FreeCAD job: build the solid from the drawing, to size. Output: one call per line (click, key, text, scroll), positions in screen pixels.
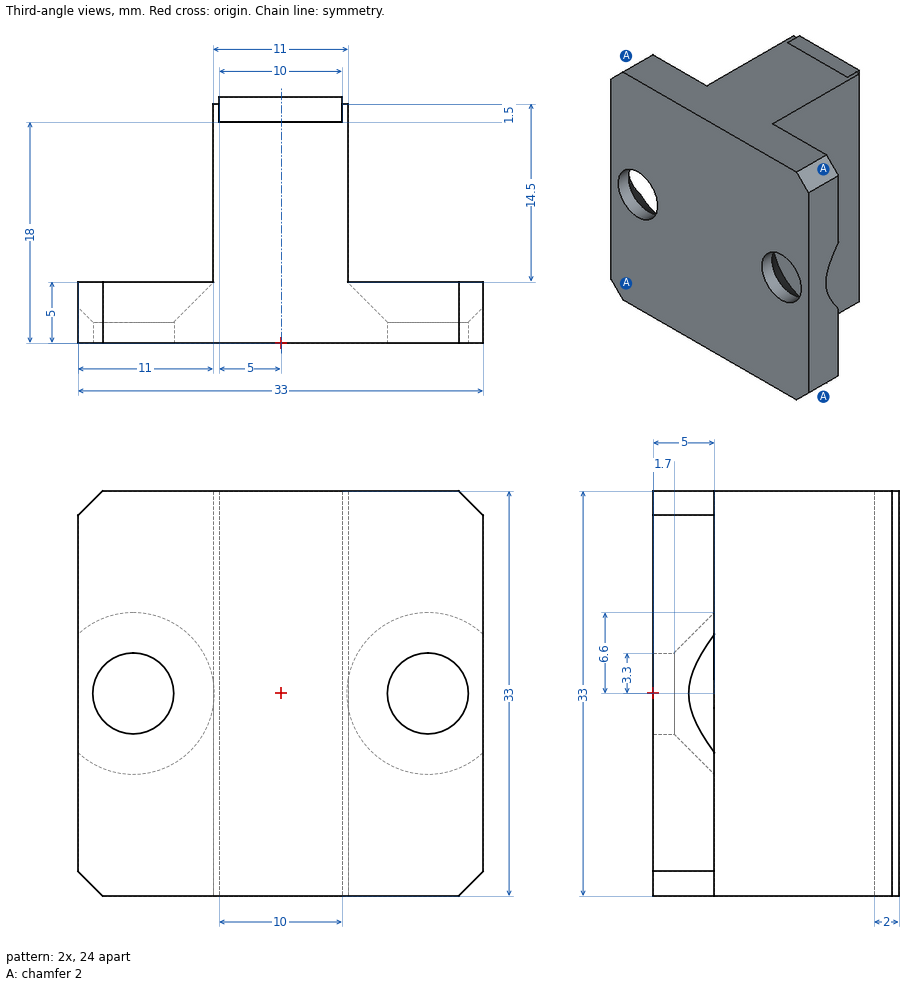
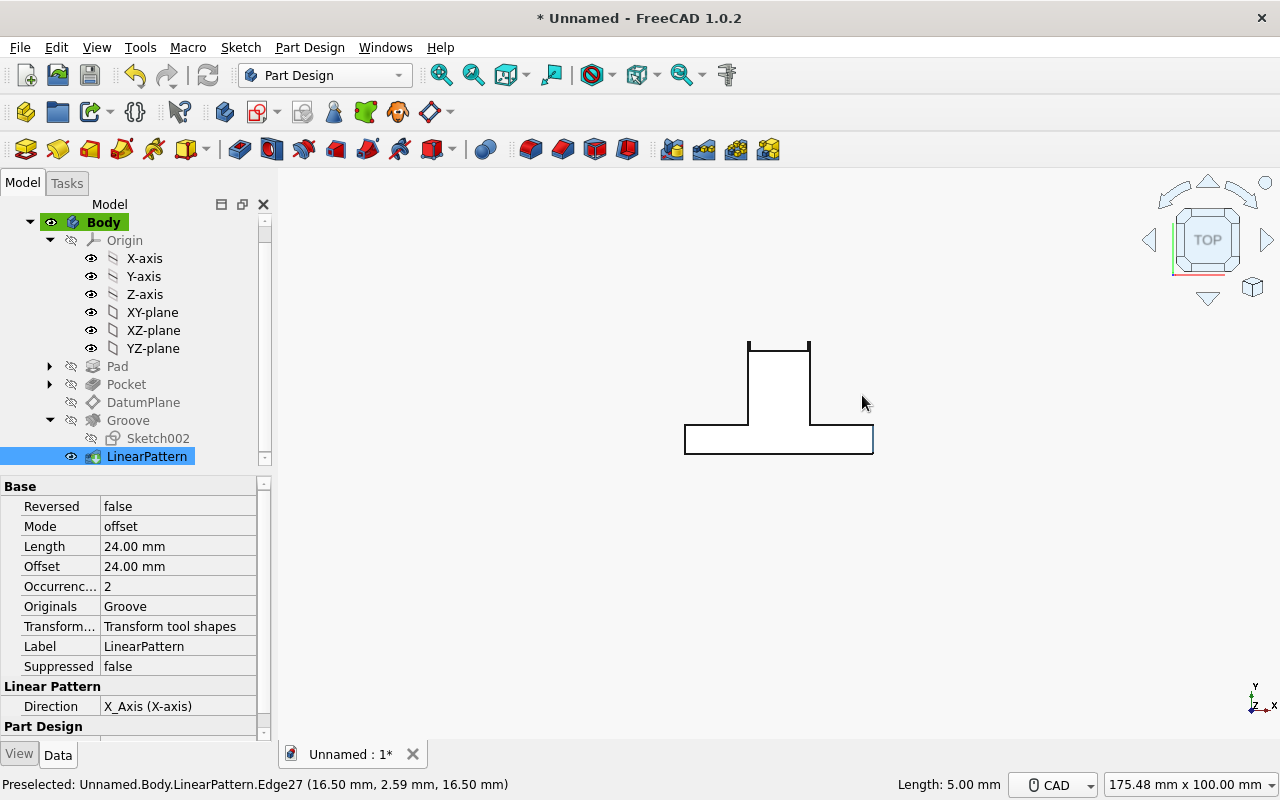
click(442, 76)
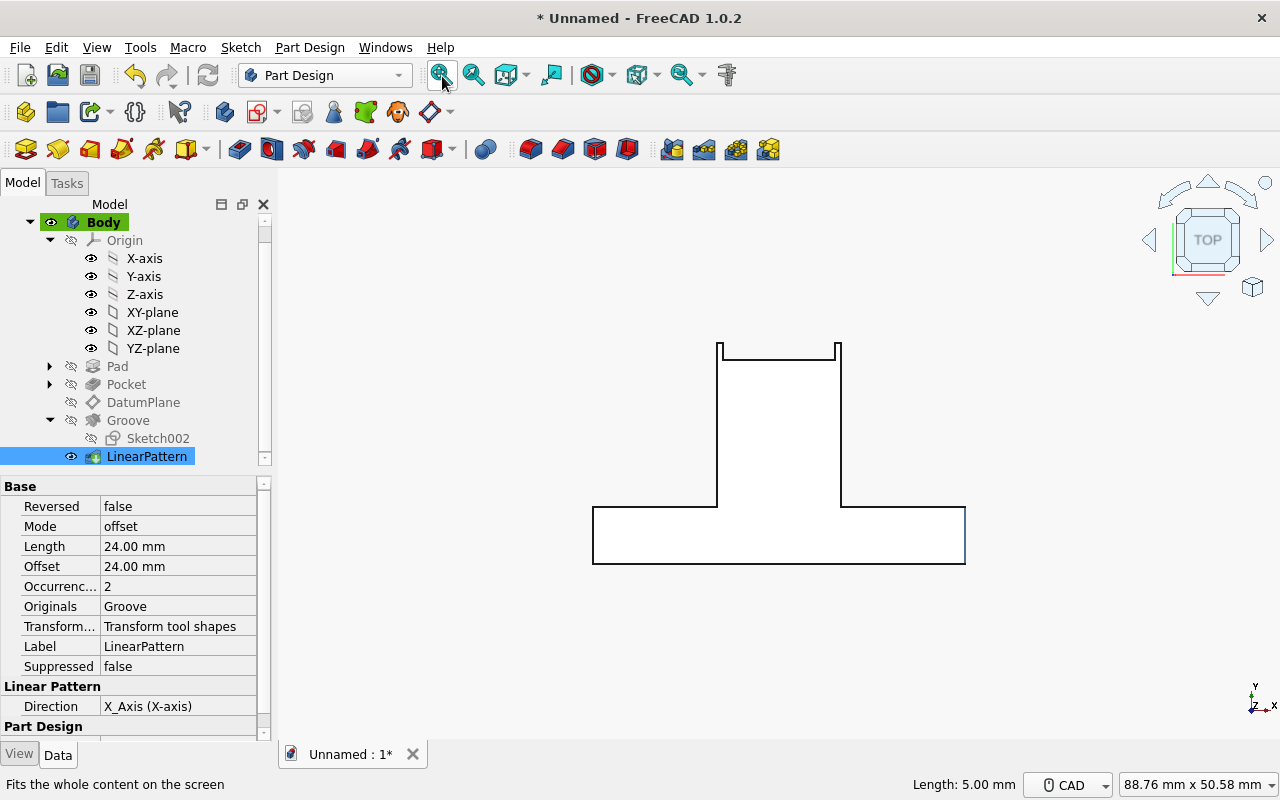
click(593, 534, ctrl)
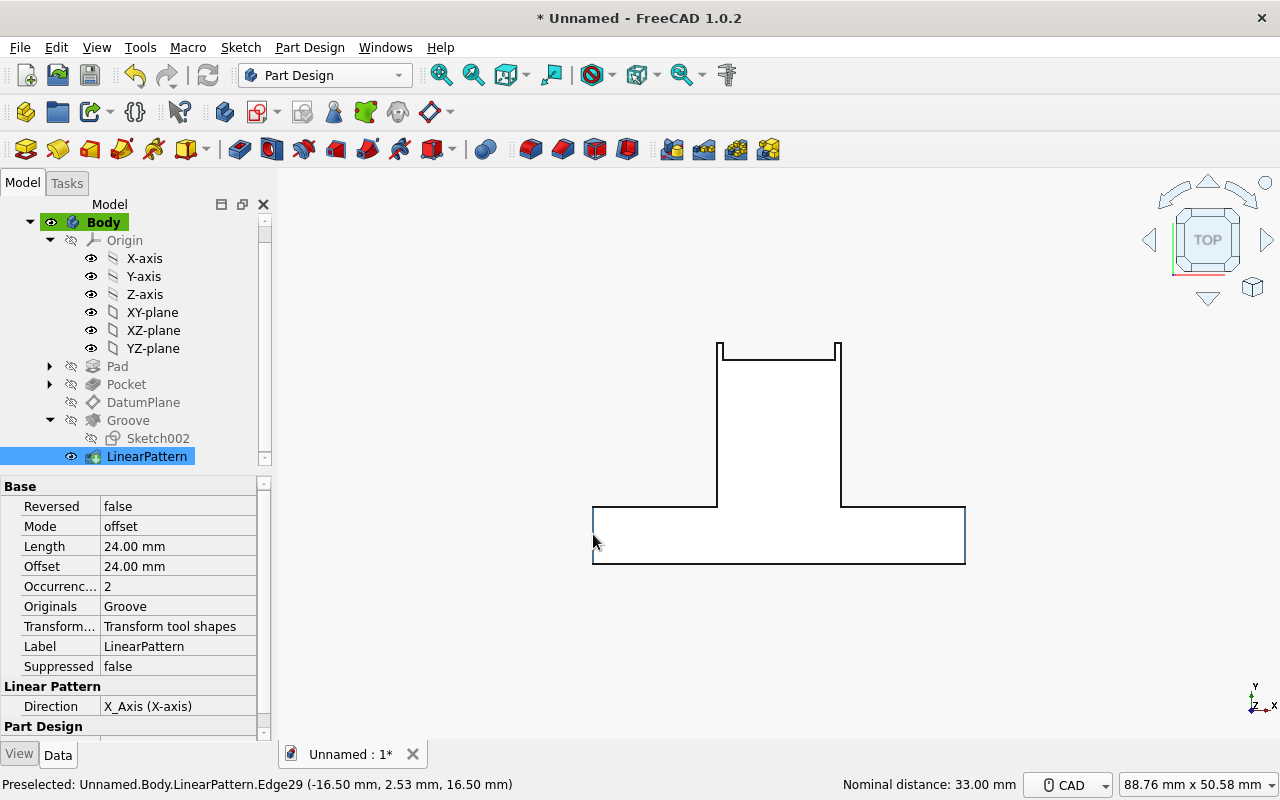
key(1)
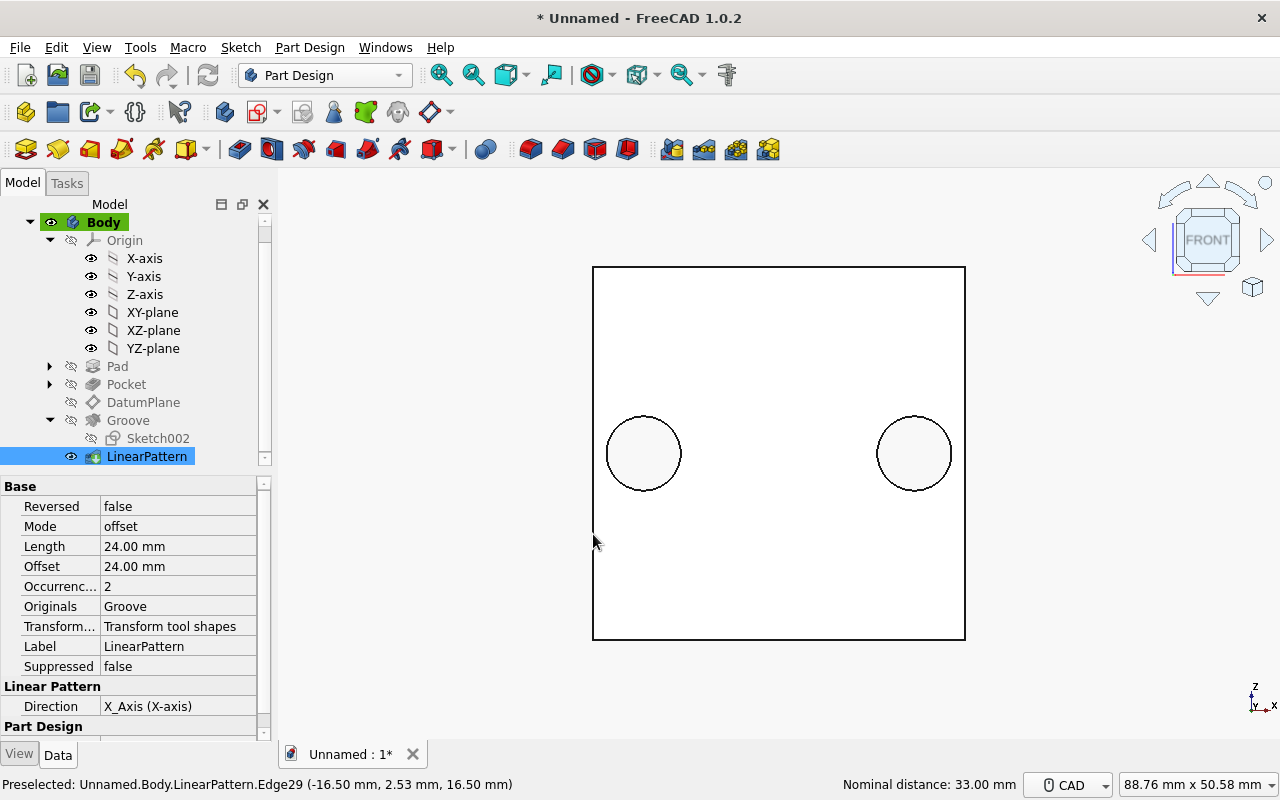
key(3)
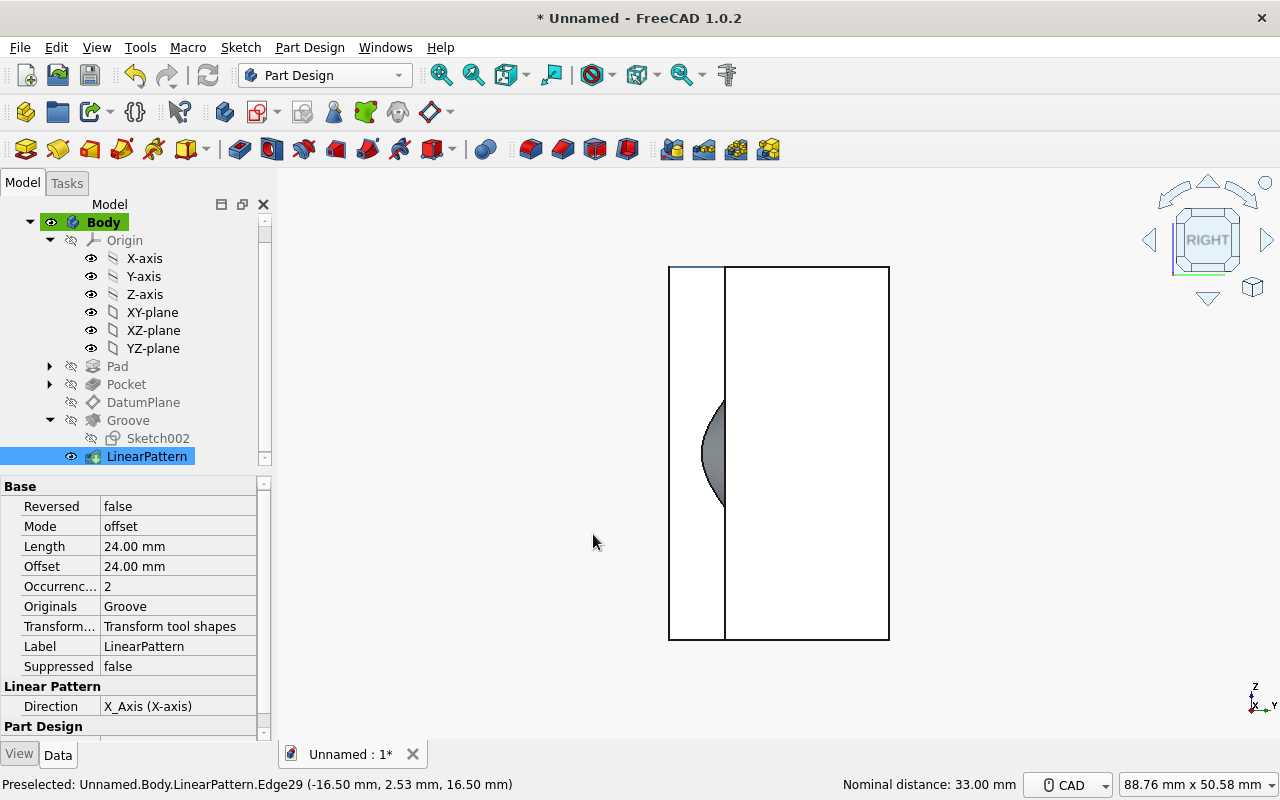
click(697, 639, ctrl)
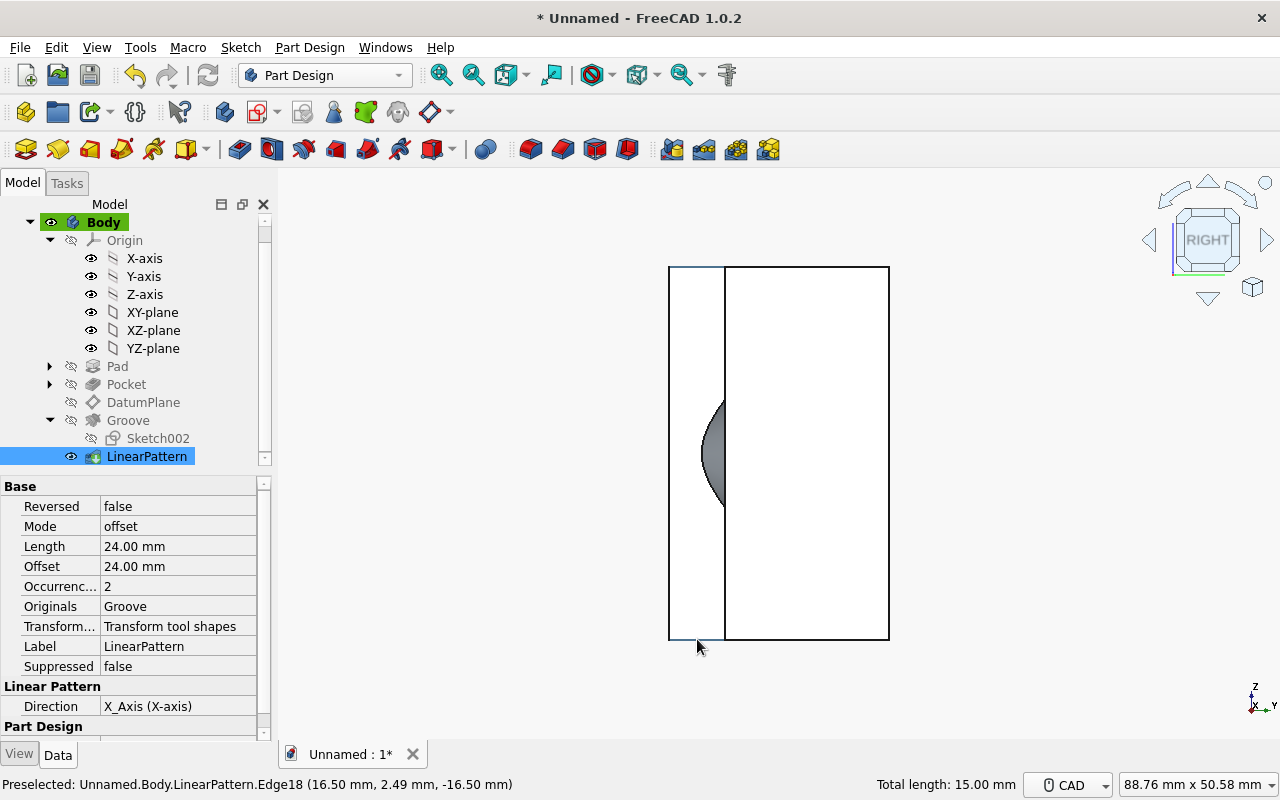
key(5)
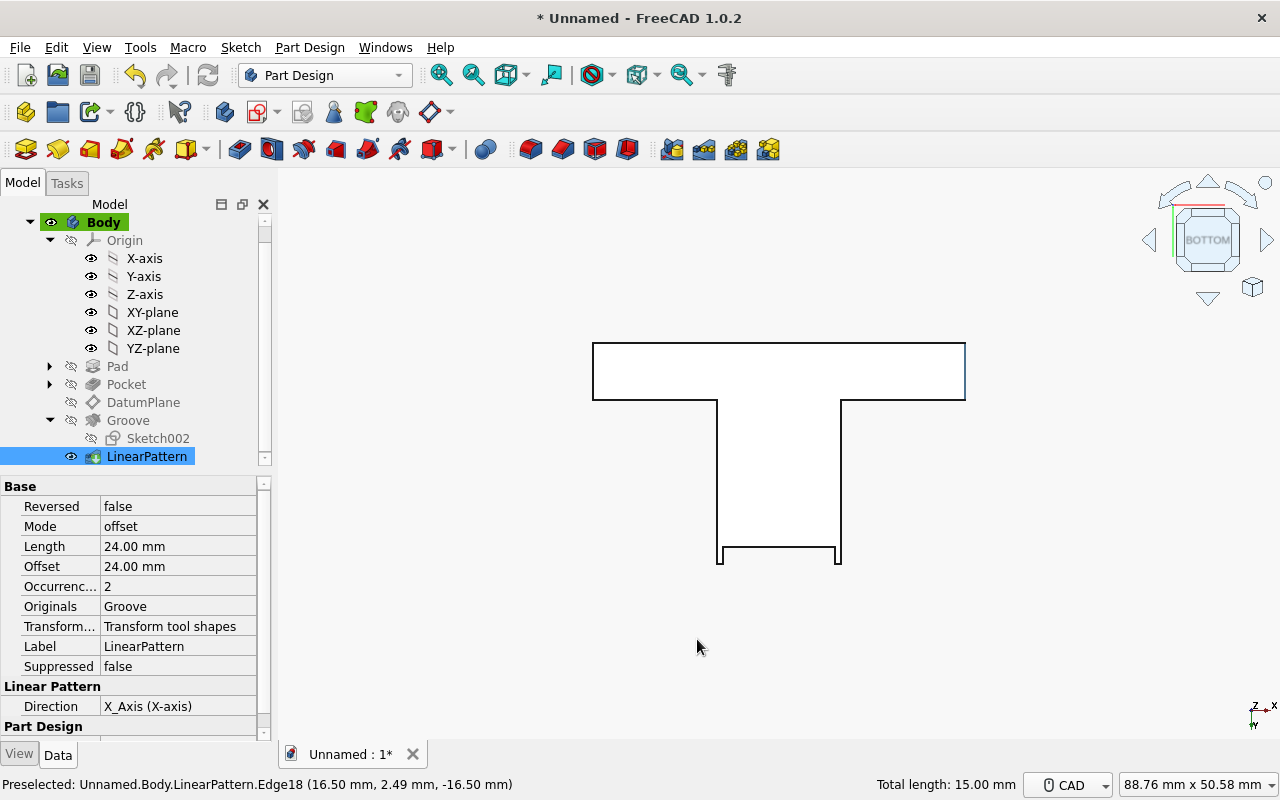
key(v)
key(f)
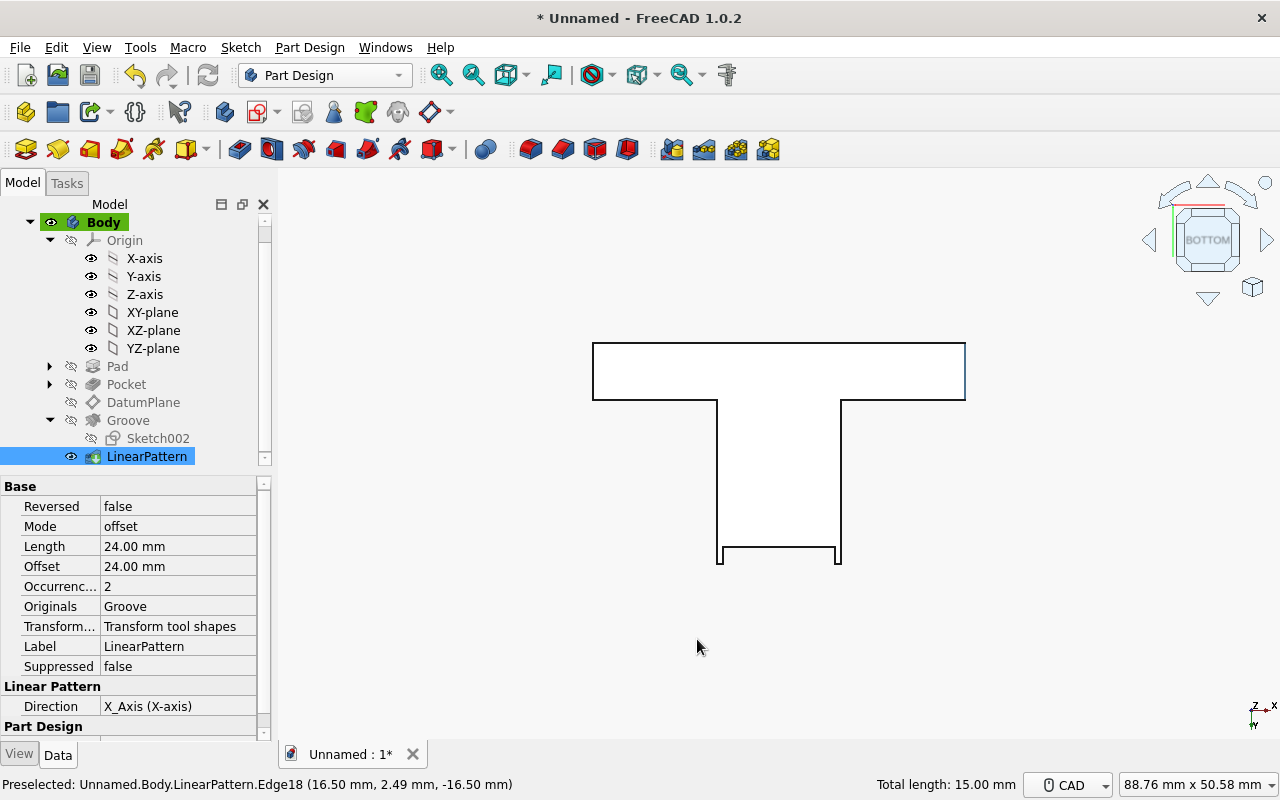
click(593, 371, ctrl)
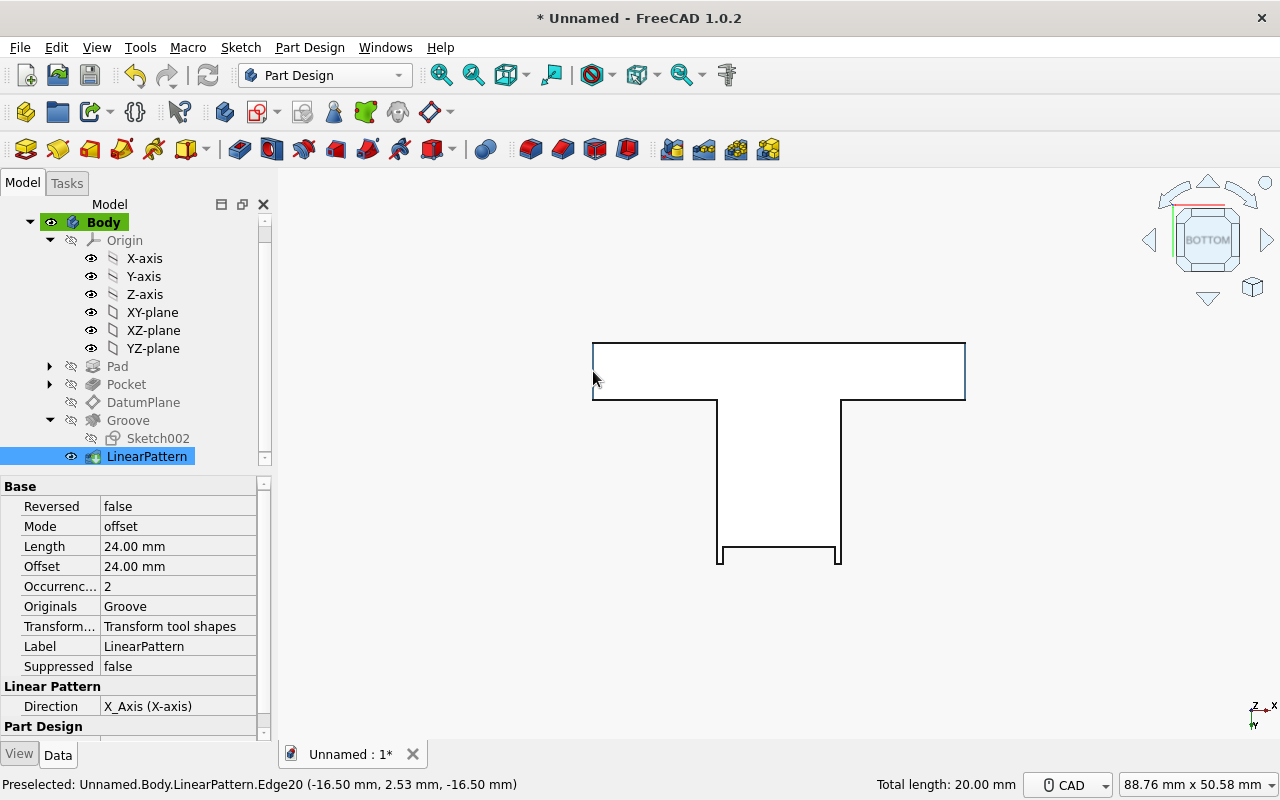
click(564, 150)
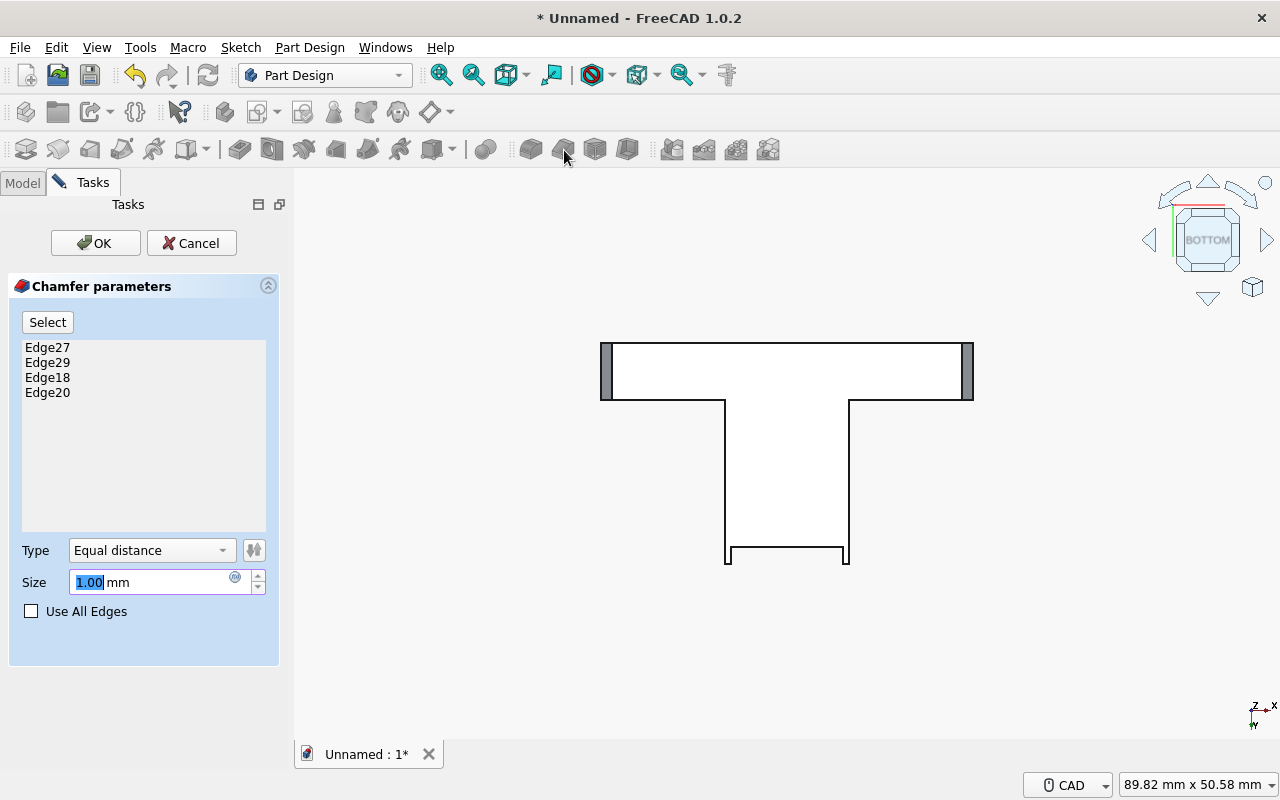
text(2)
key(Tab)